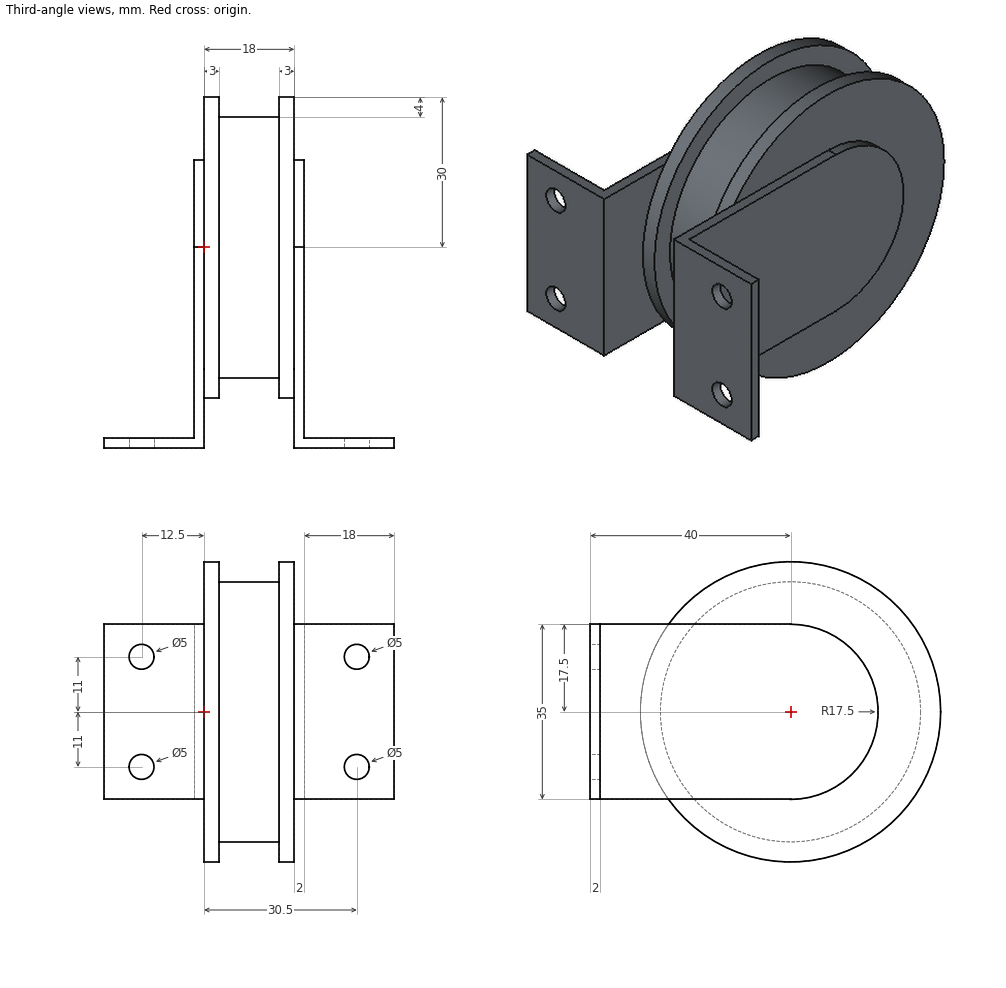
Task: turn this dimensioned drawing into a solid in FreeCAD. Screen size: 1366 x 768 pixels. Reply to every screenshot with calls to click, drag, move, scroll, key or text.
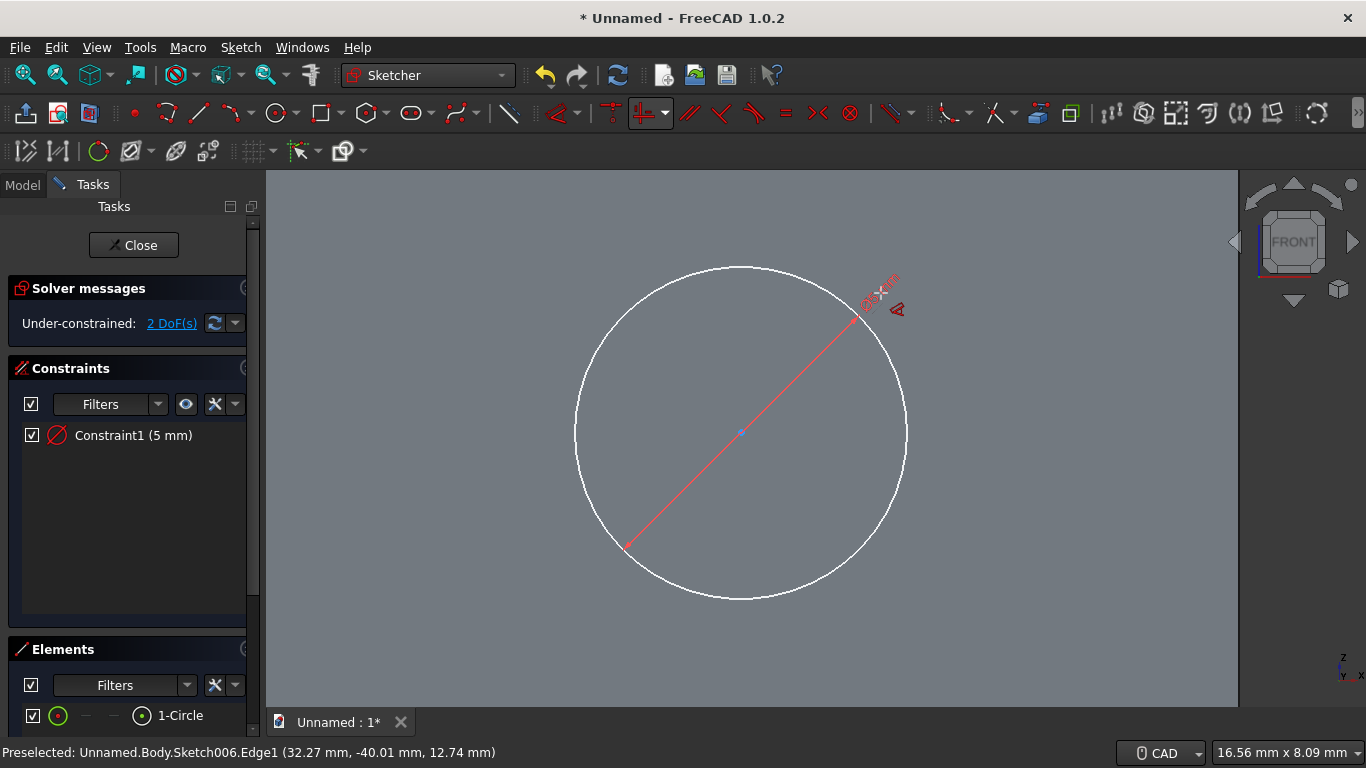
click(741, 433)
click(775, 556)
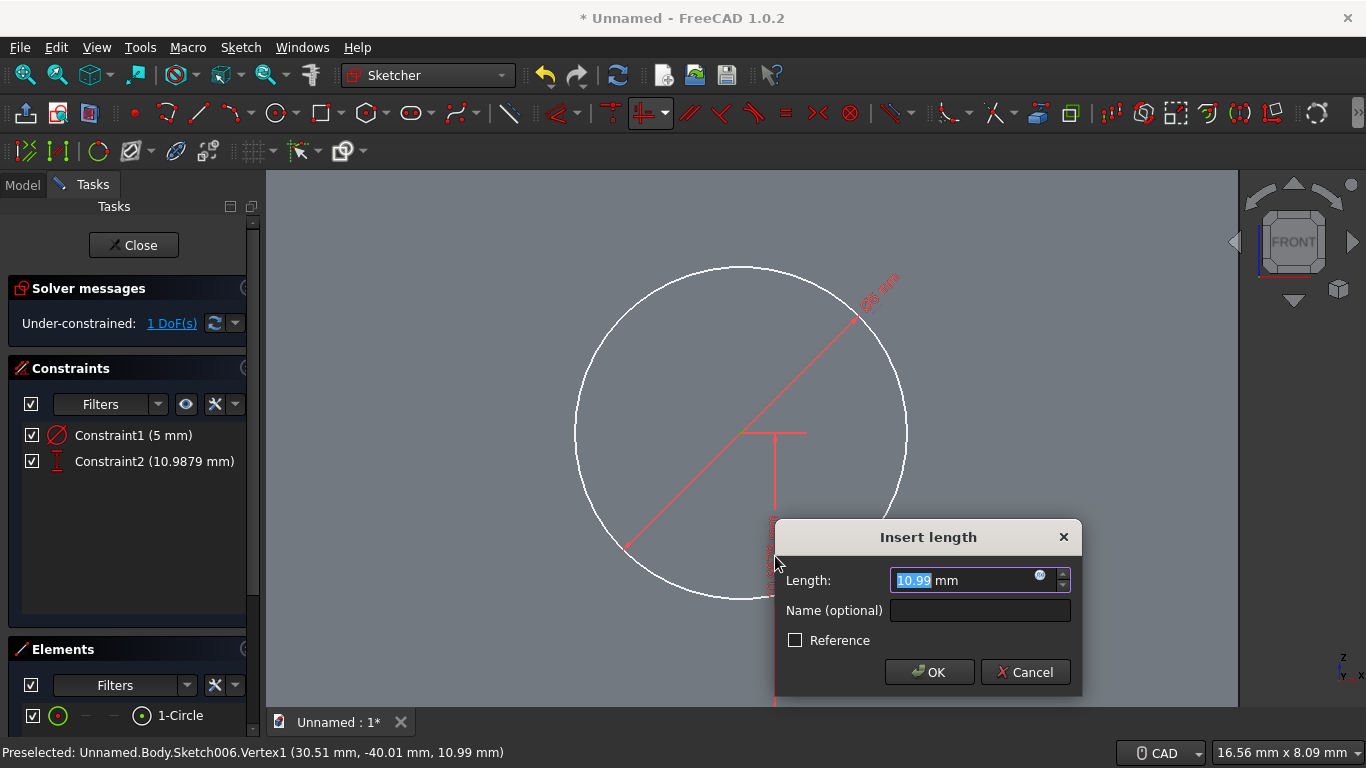
text(11)
key(Return)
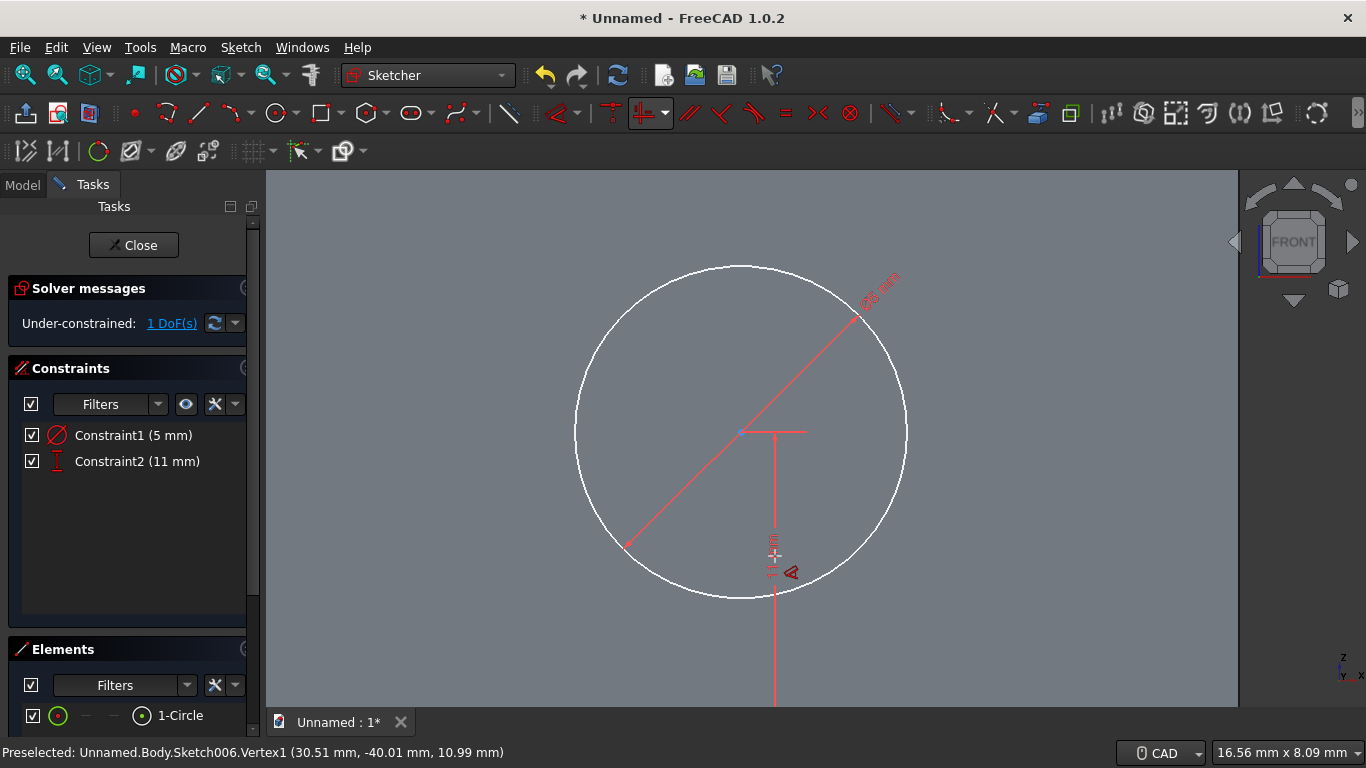
click(741, 432)
click(518, 398)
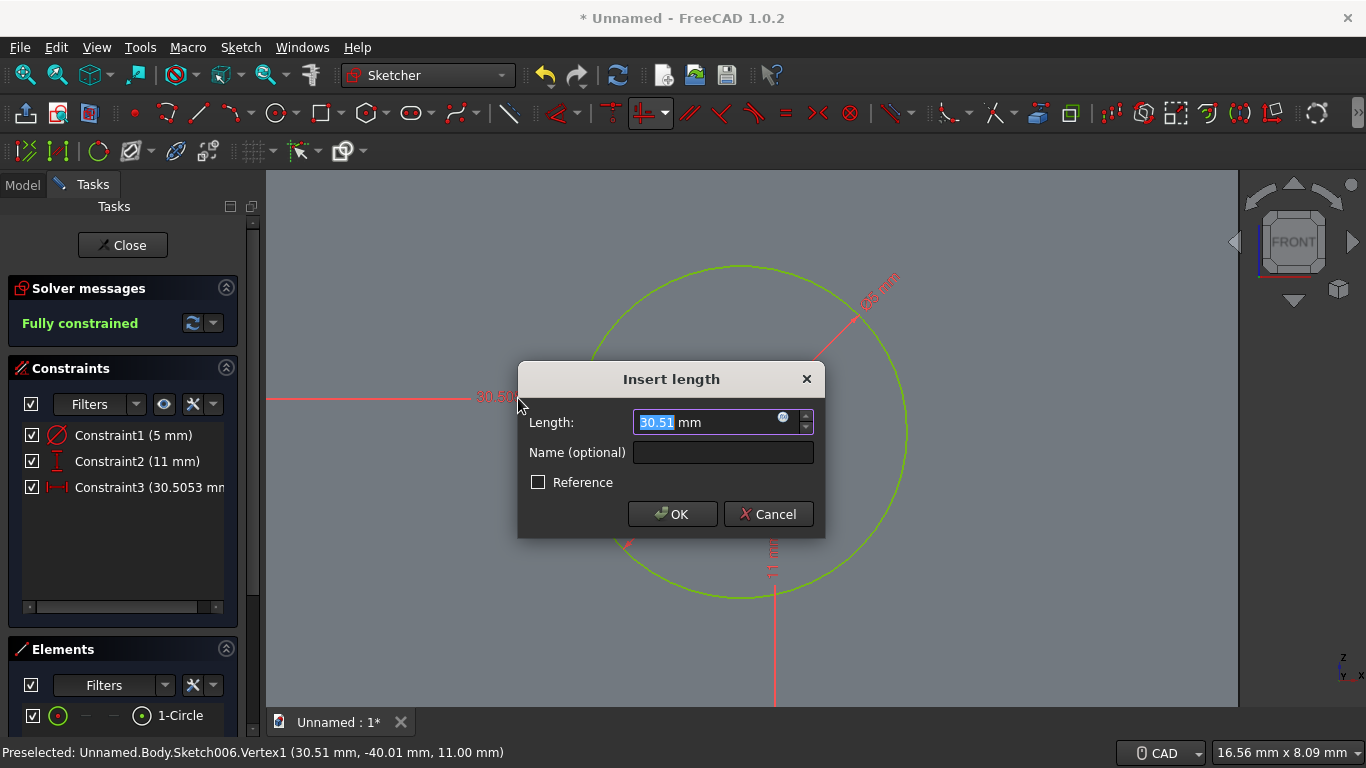
text(30.5)
key(Return)
key(Escape)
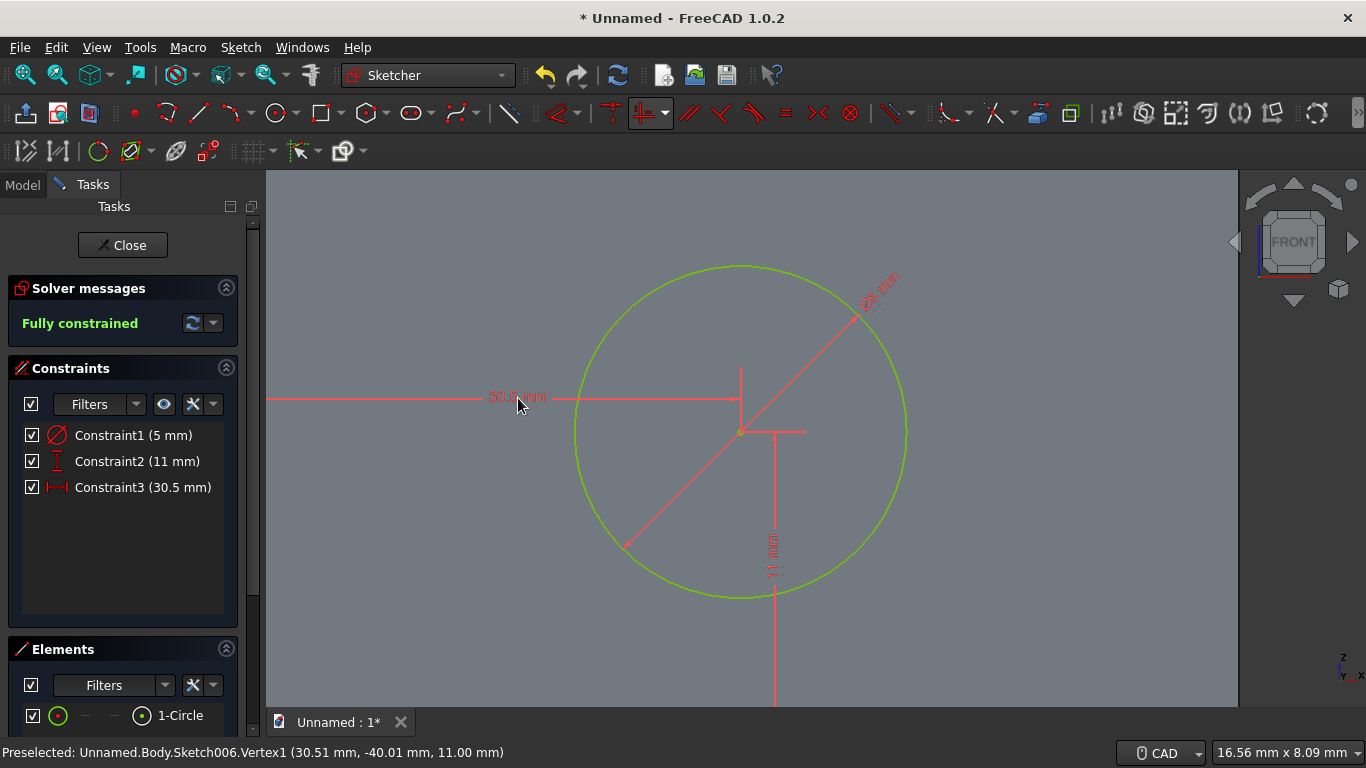
click(123, 245)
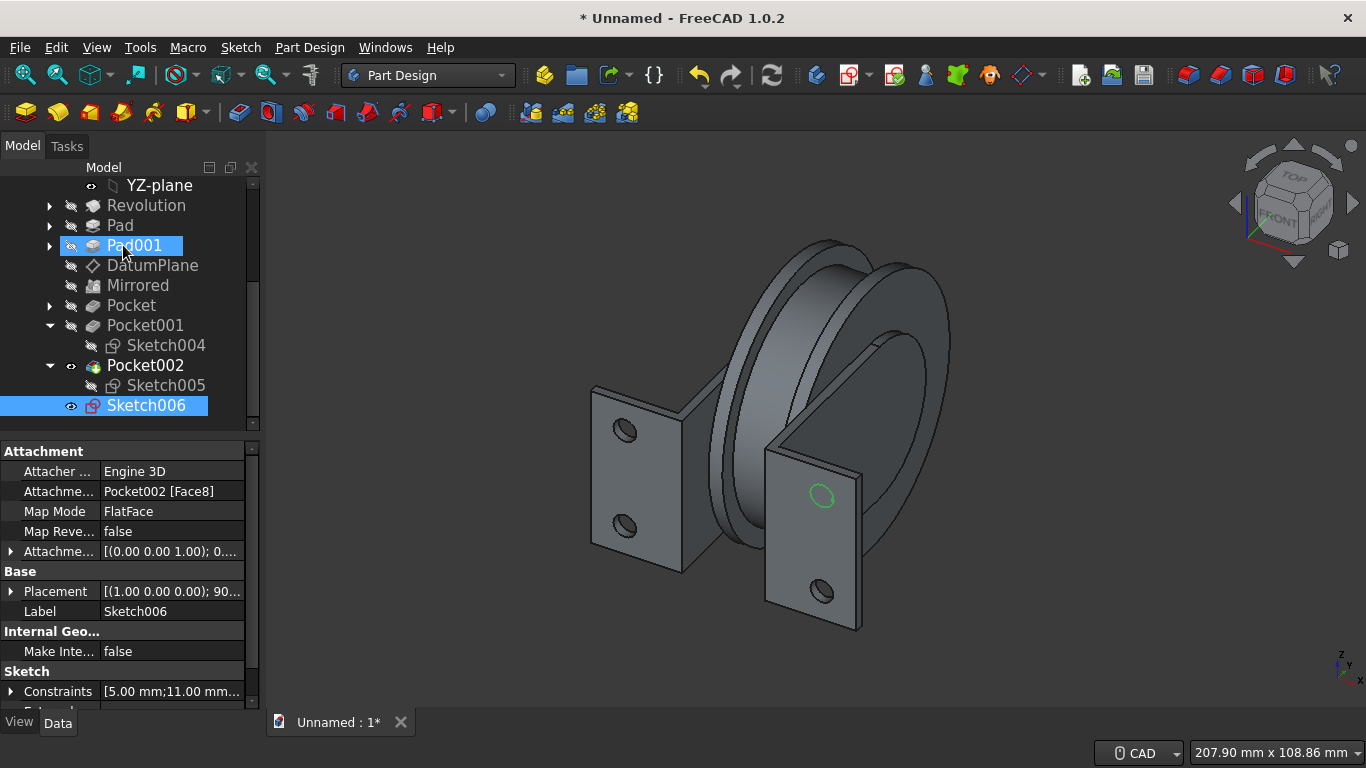
click(240, 112)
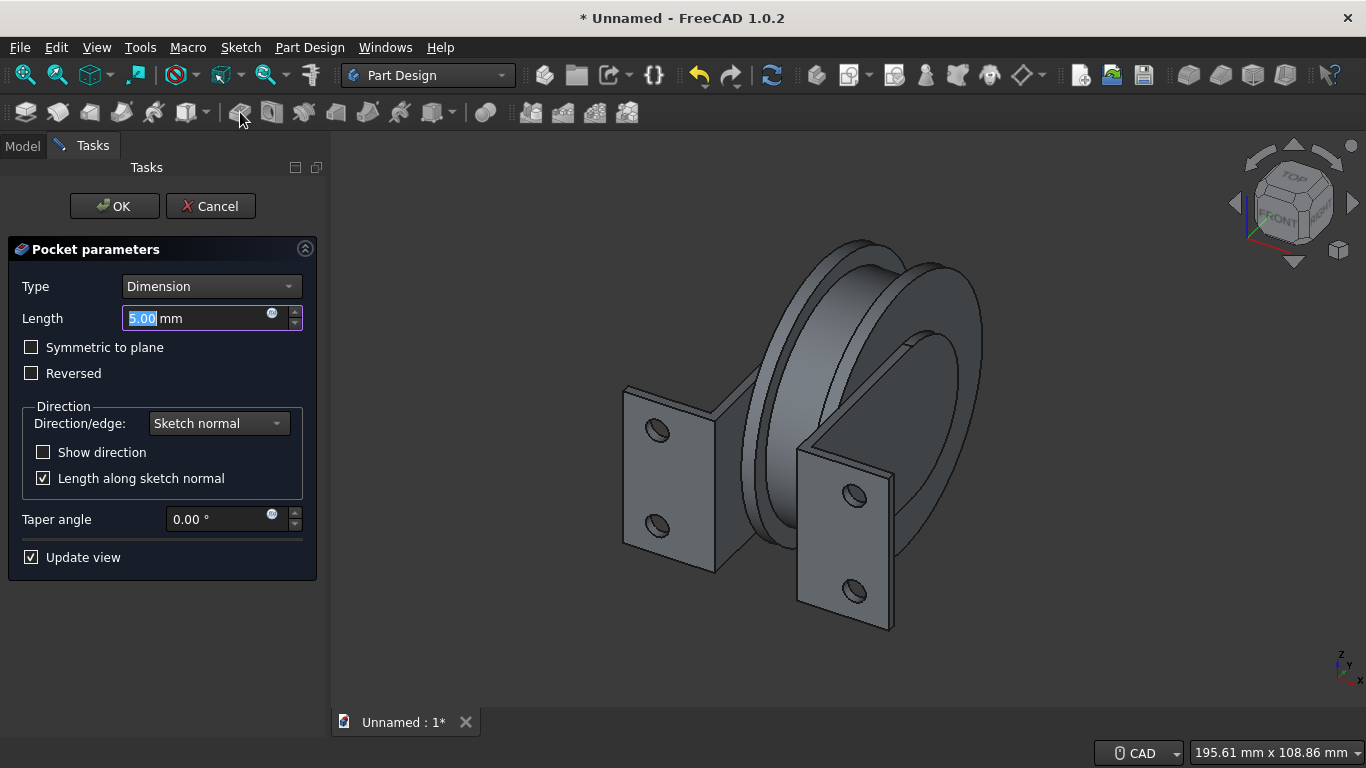
click(212, 286)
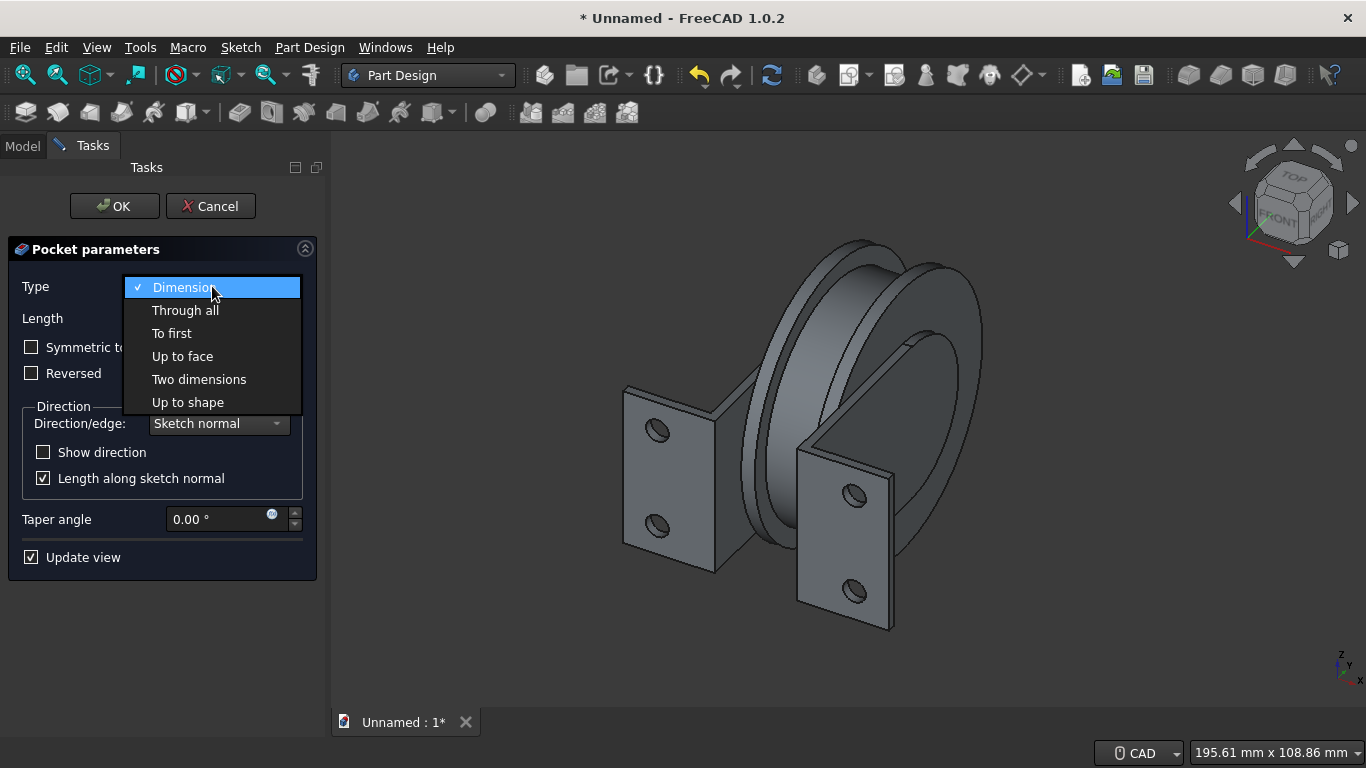
click(212, 334)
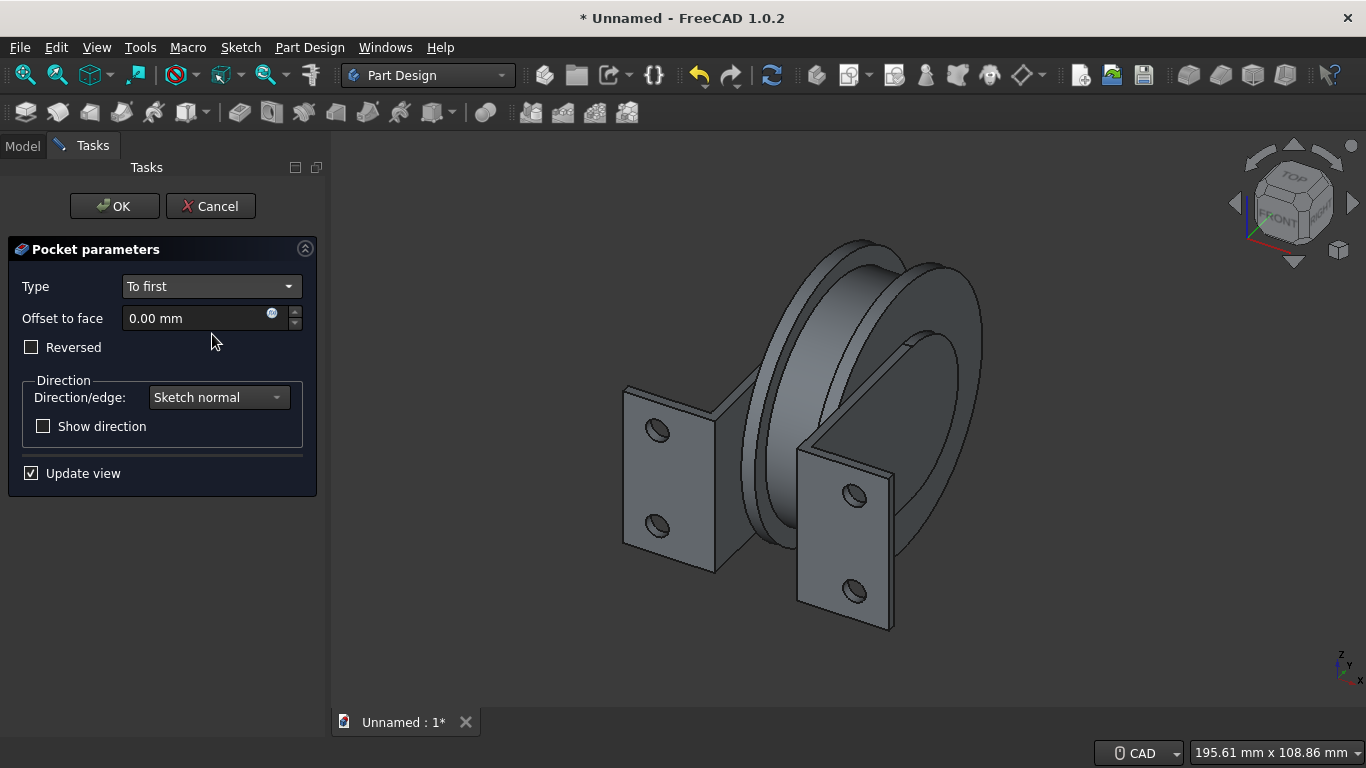
click(115, 206)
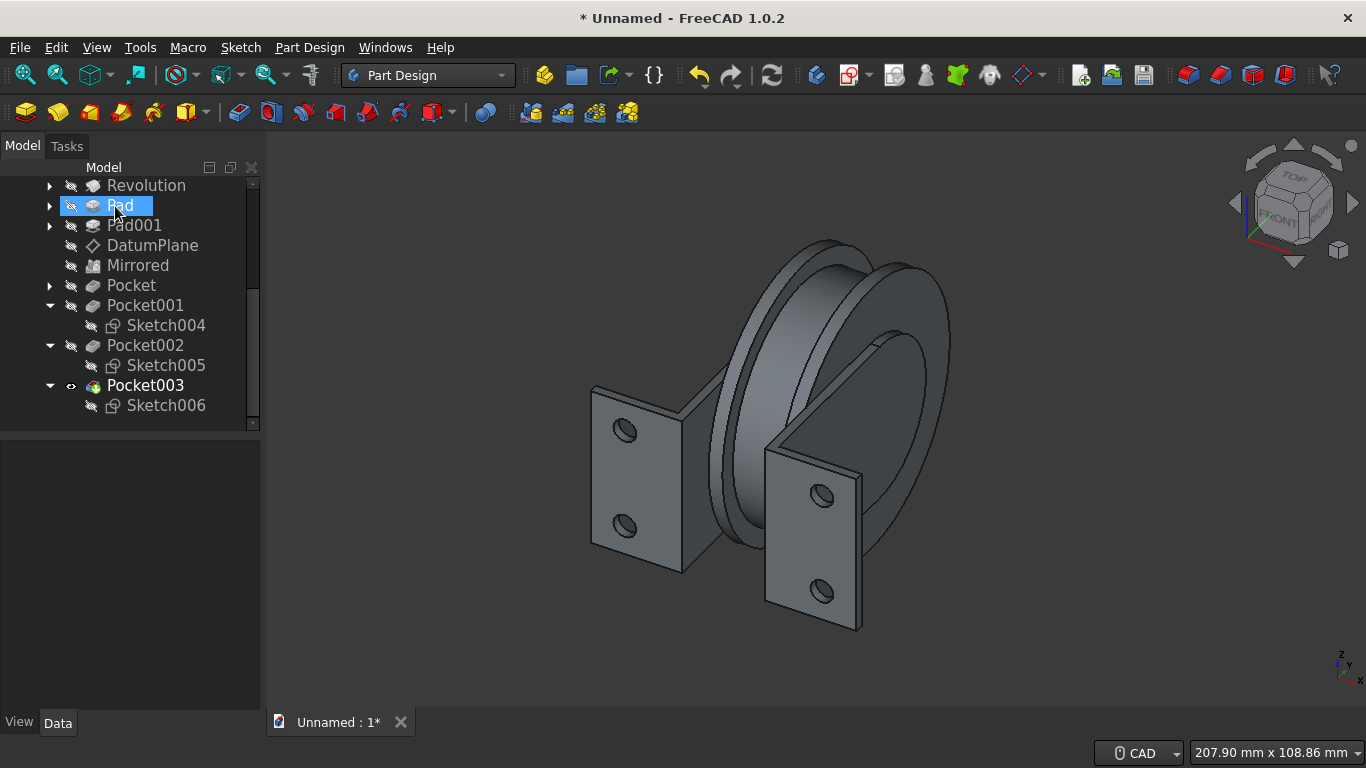
key(0)